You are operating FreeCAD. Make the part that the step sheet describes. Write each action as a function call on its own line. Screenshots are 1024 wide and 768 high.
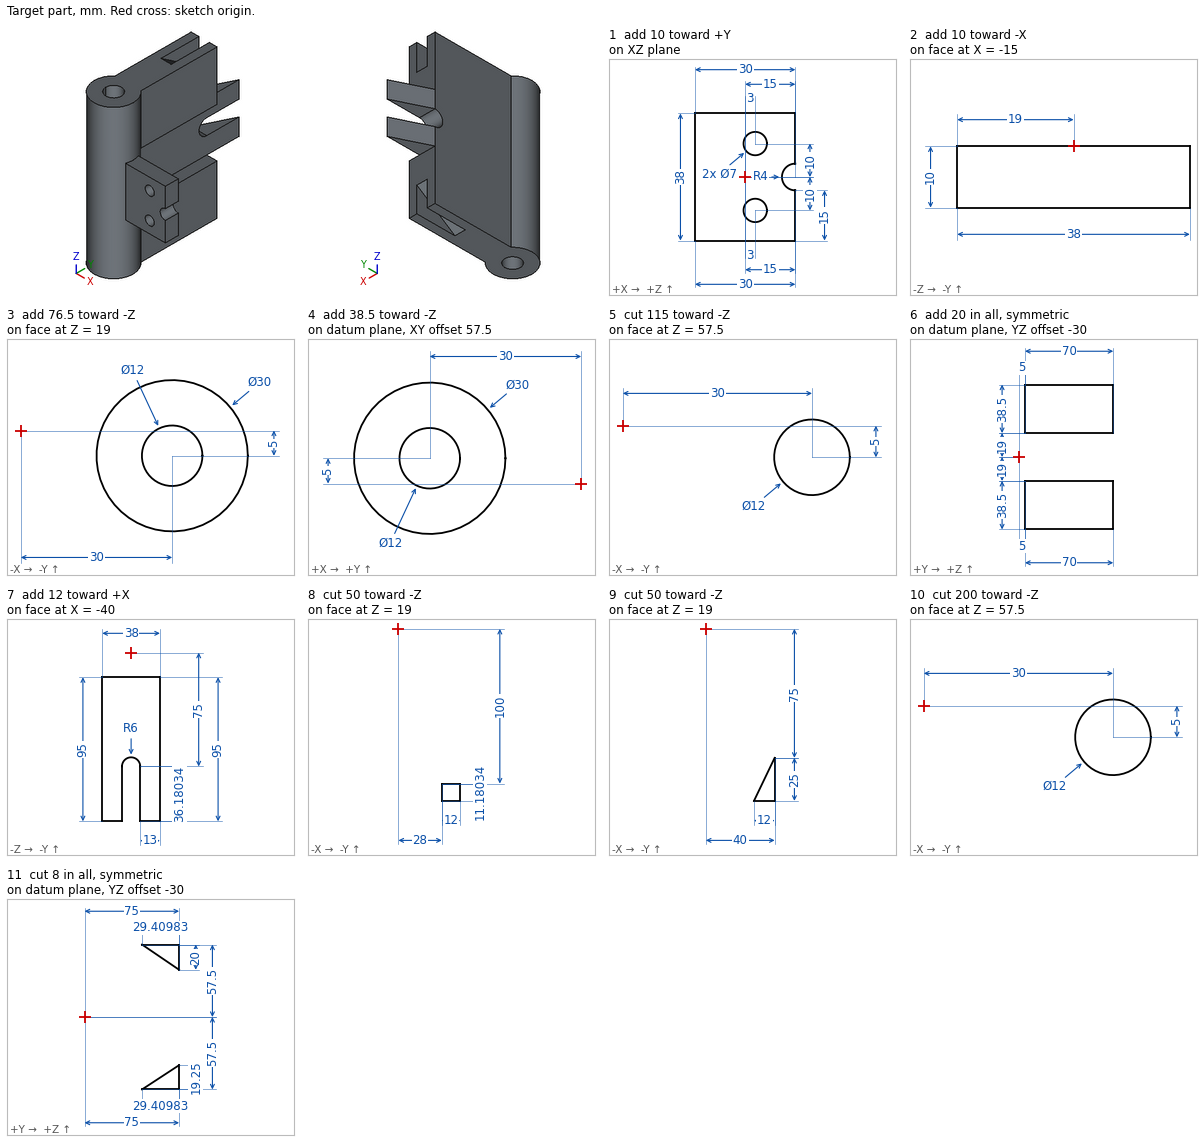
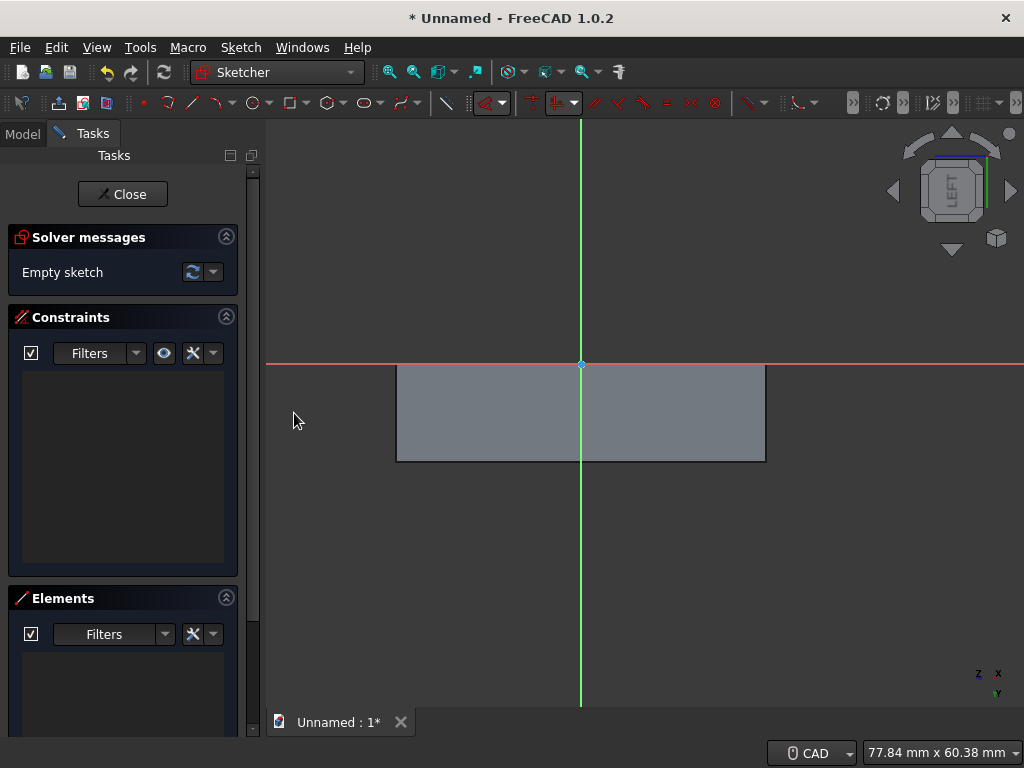
key(g)
key(r)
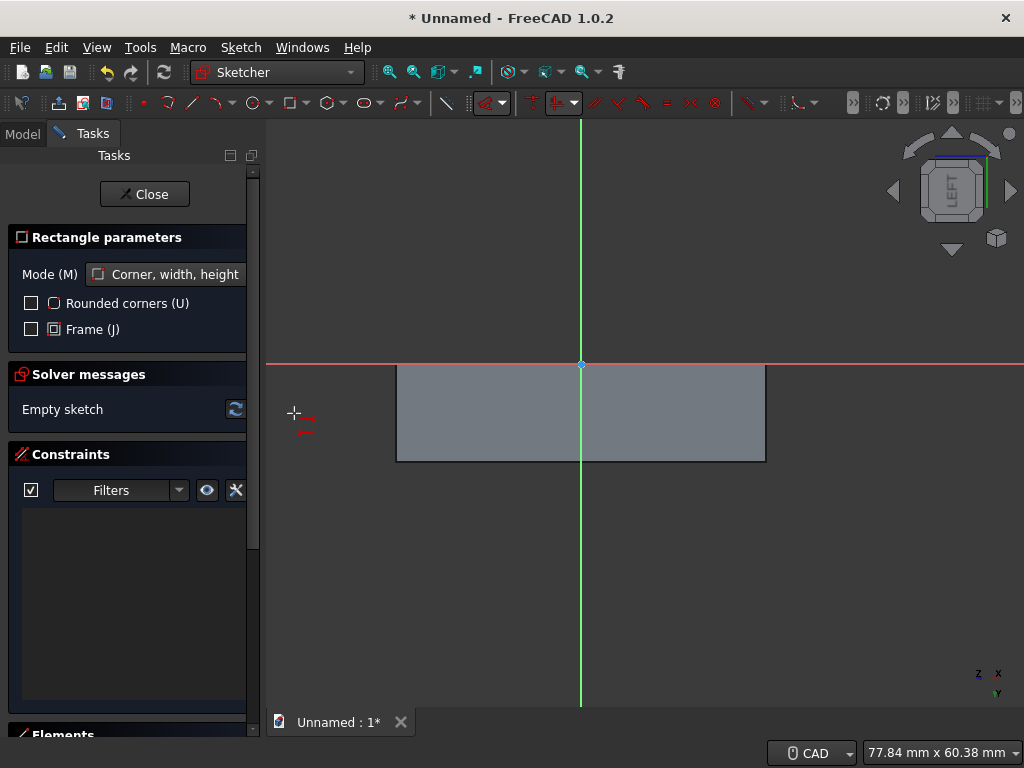
click(396, 364)
click(766, 462)
key(Escape)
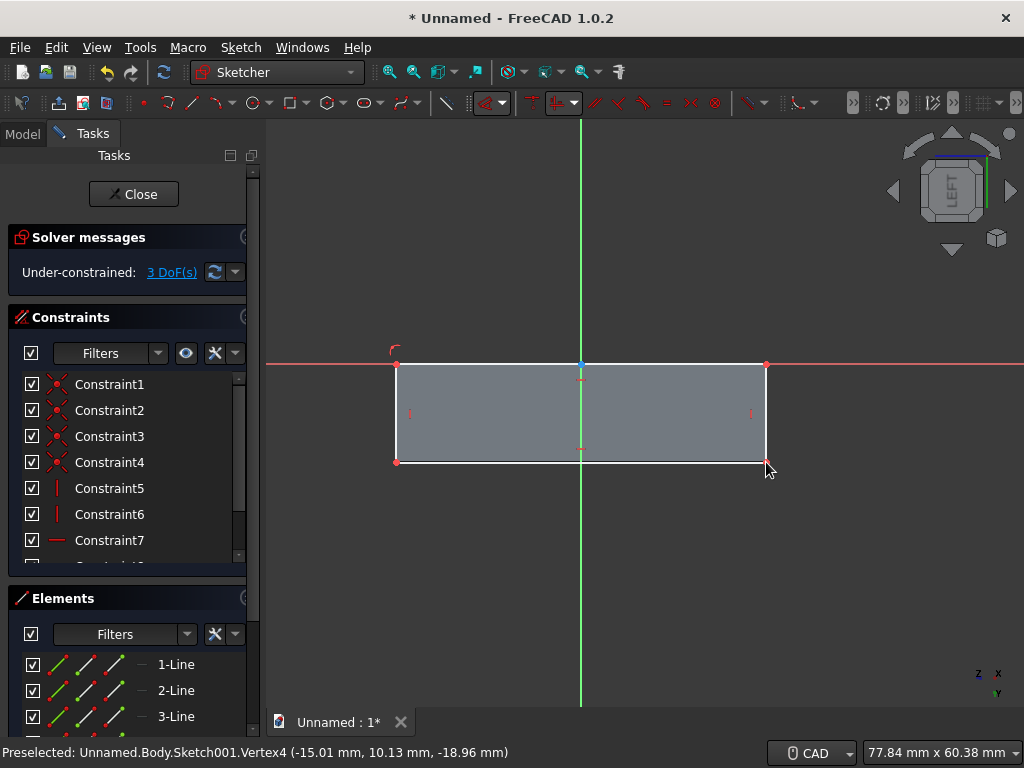
click(396, 394)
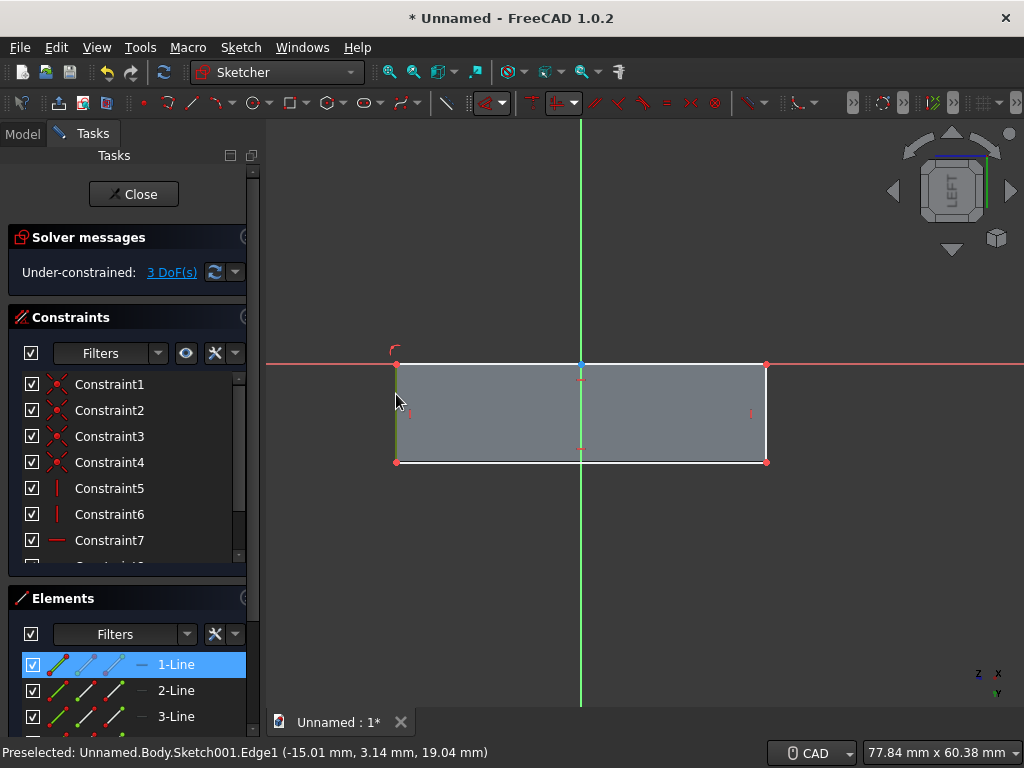
click(504, 104)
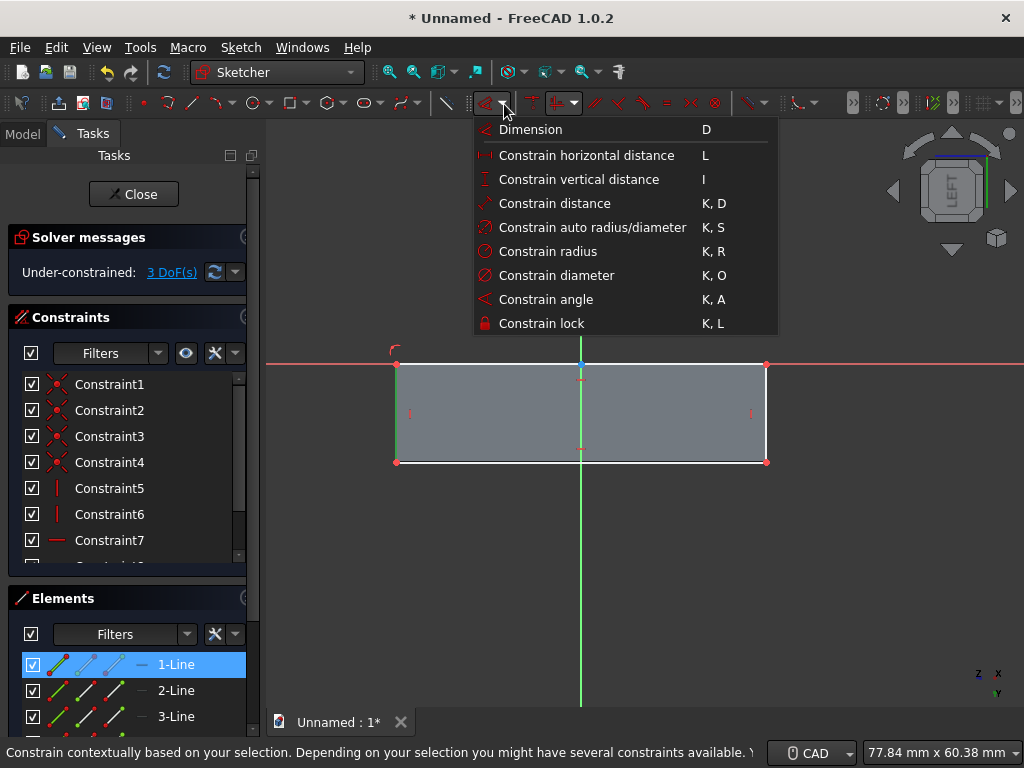
click(626, 179)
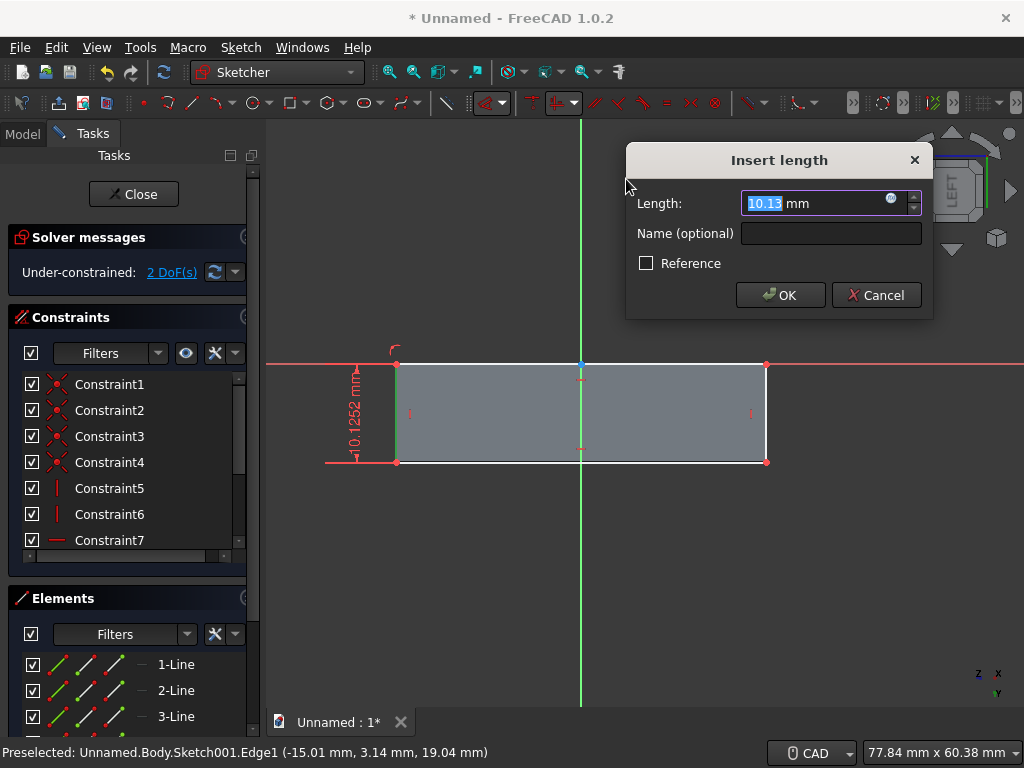
text(10)
key(Return)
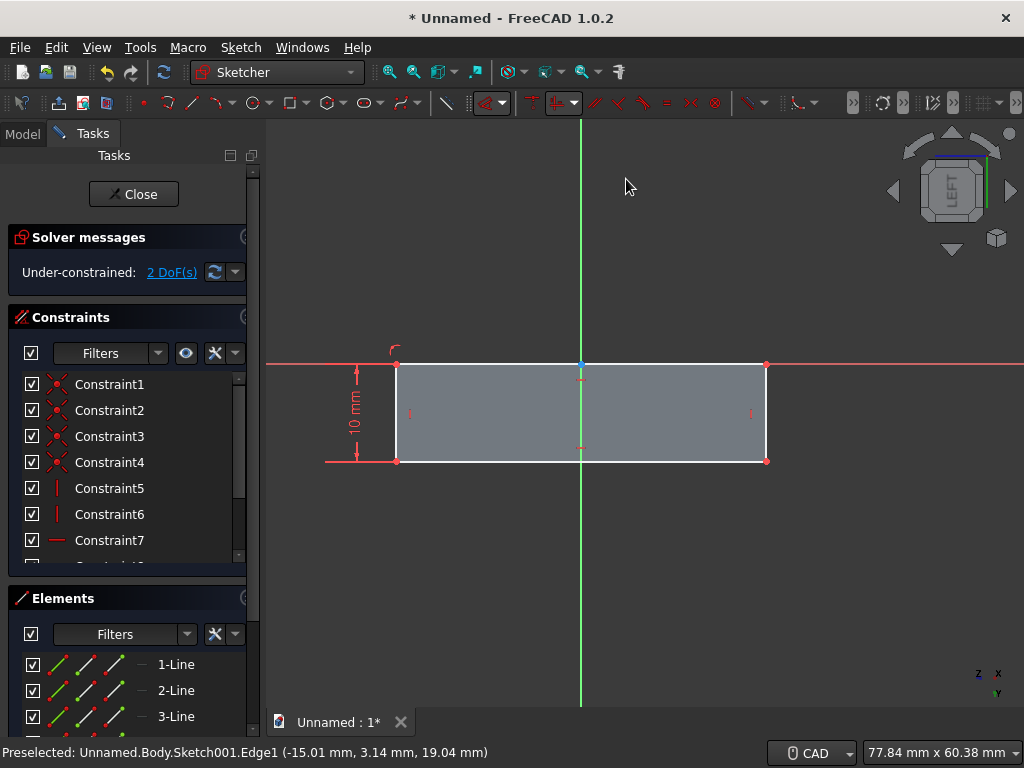
click(507, 462)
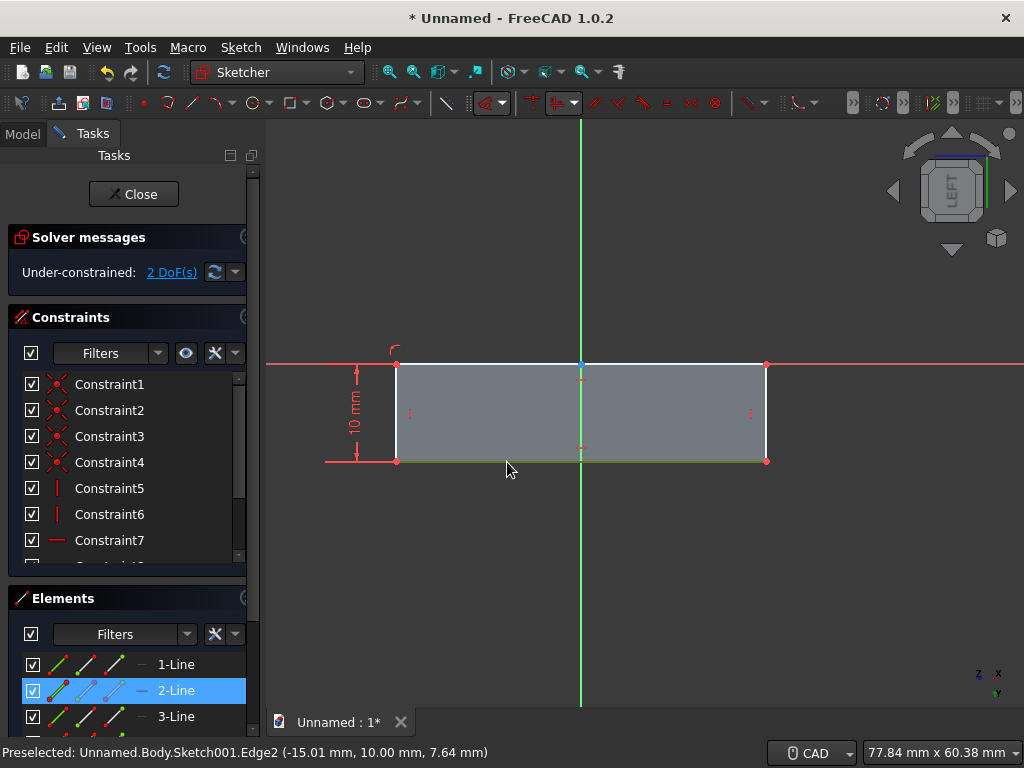
key(l)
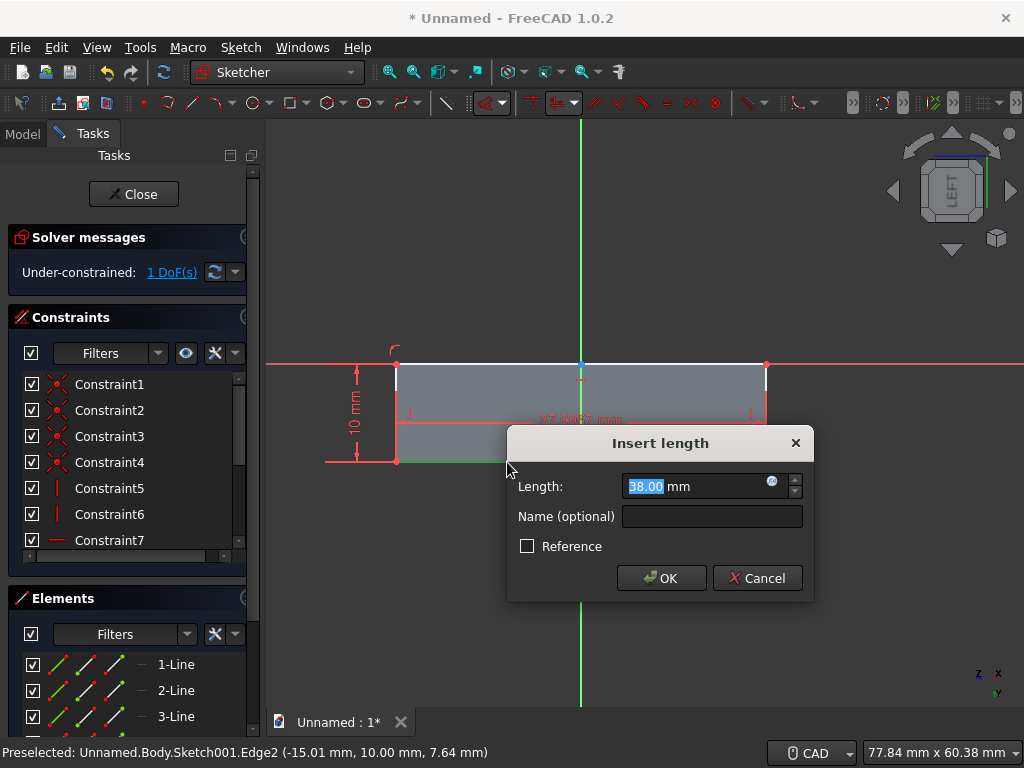
text(38)
key(Return)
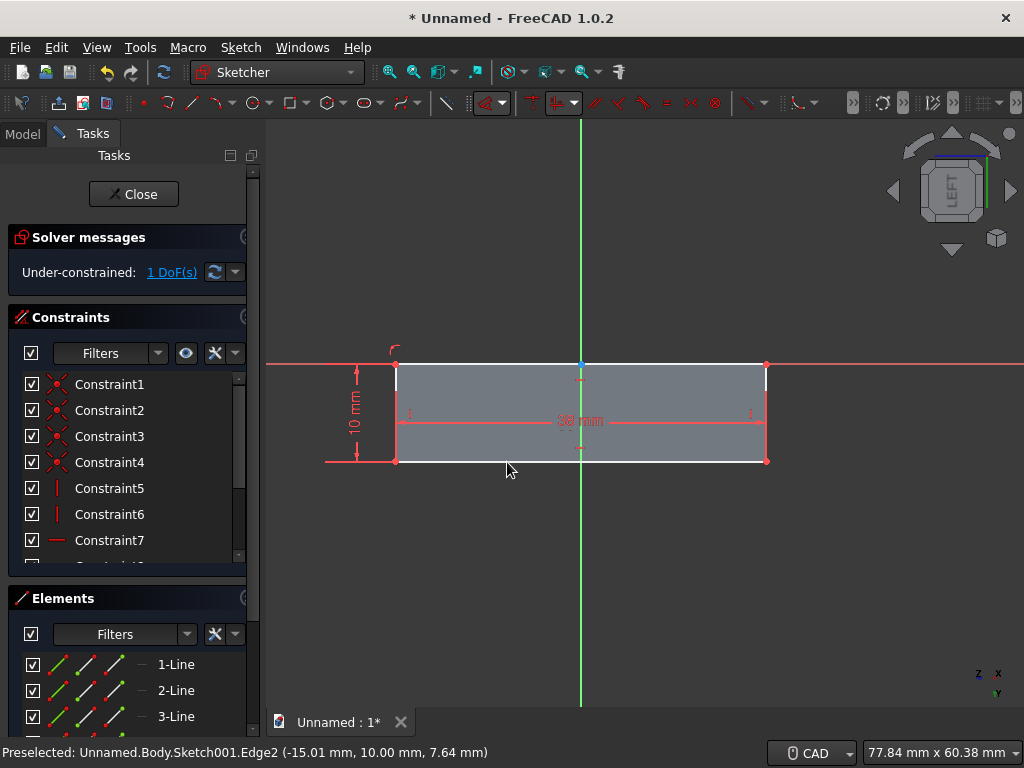
click(396, 364)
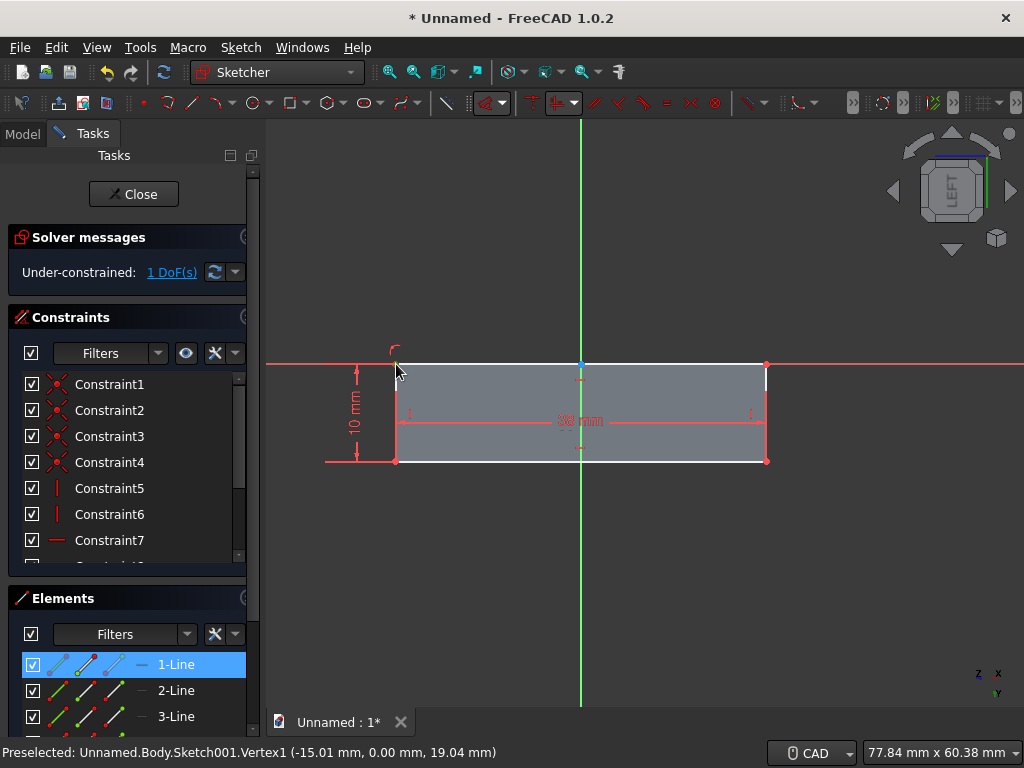
key(l)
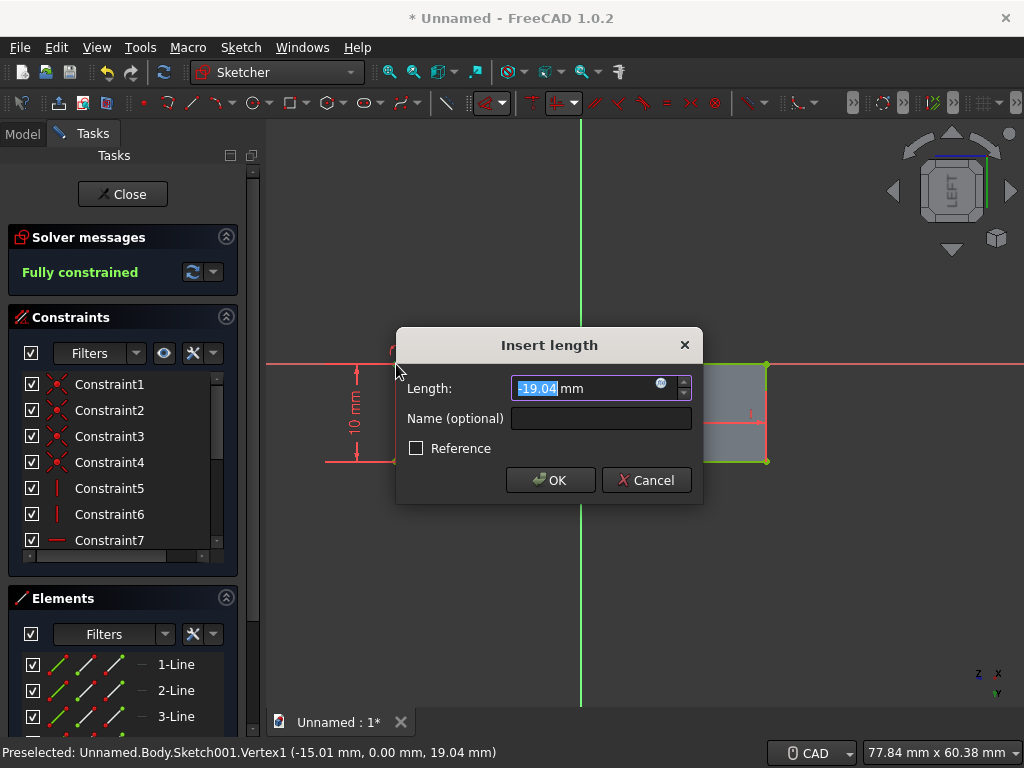
text(-19)
key(Return)